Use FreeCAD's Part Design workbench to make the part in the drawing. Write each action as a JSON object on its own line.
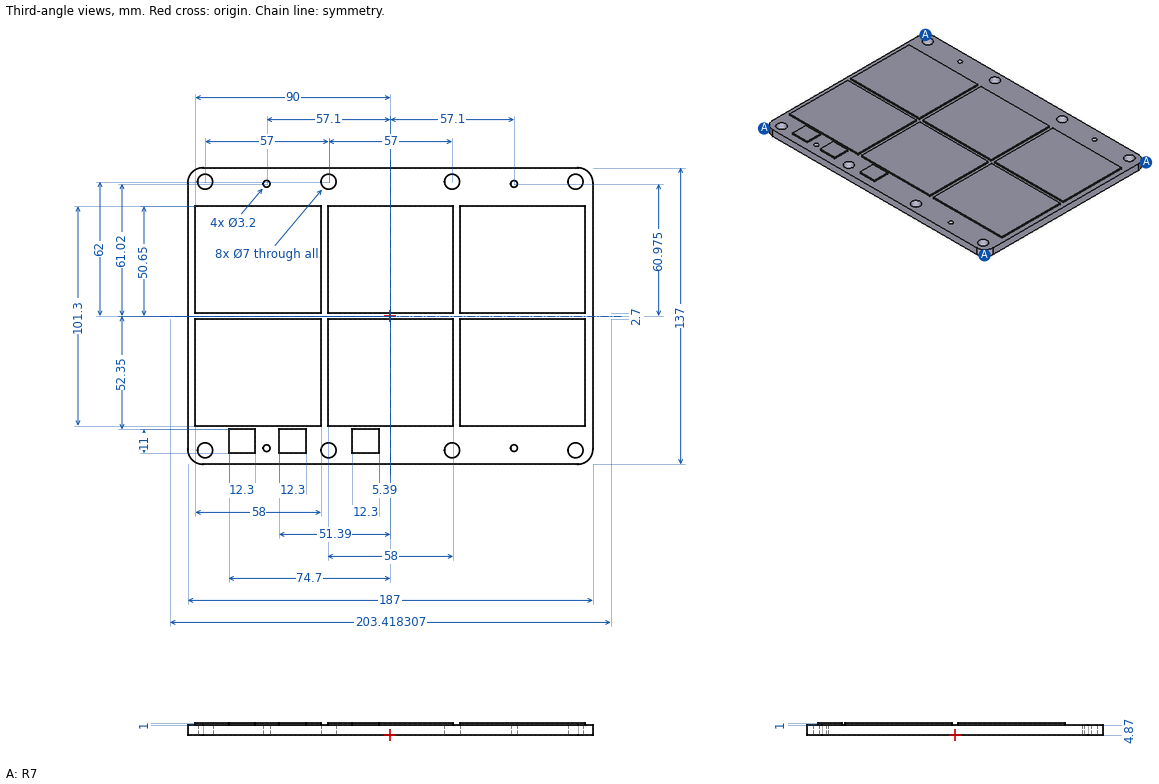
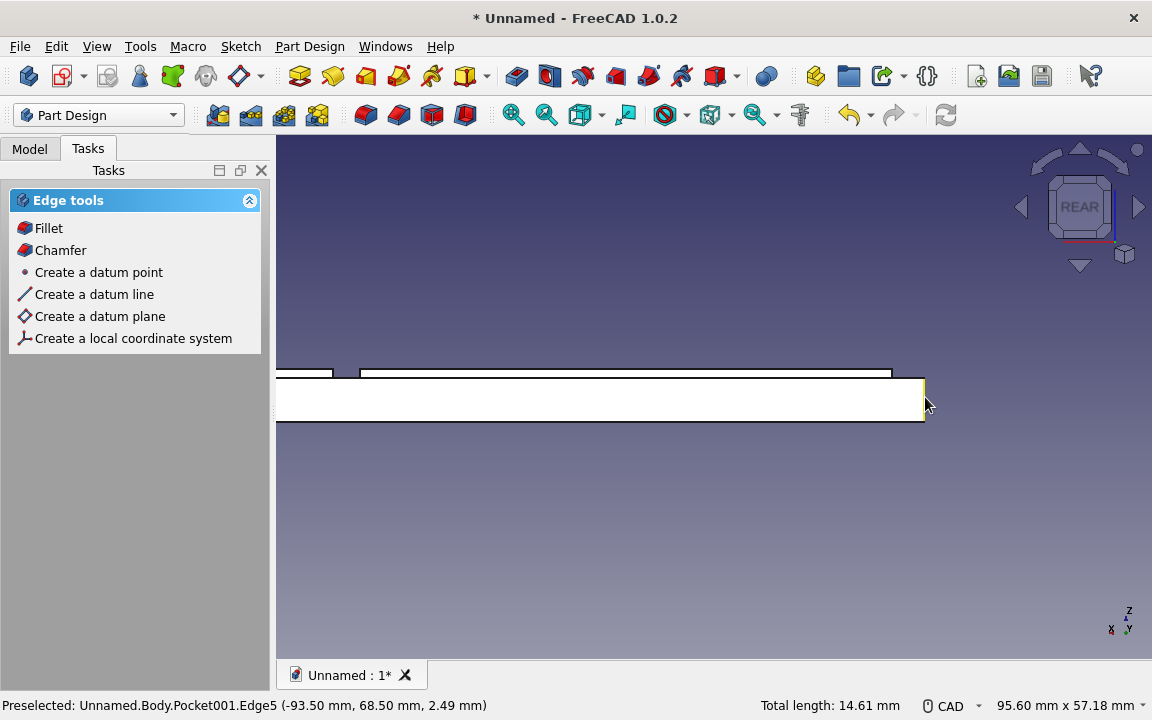
{"action": "left_click", "coordinate": [924, 399], "text": "ctrl"}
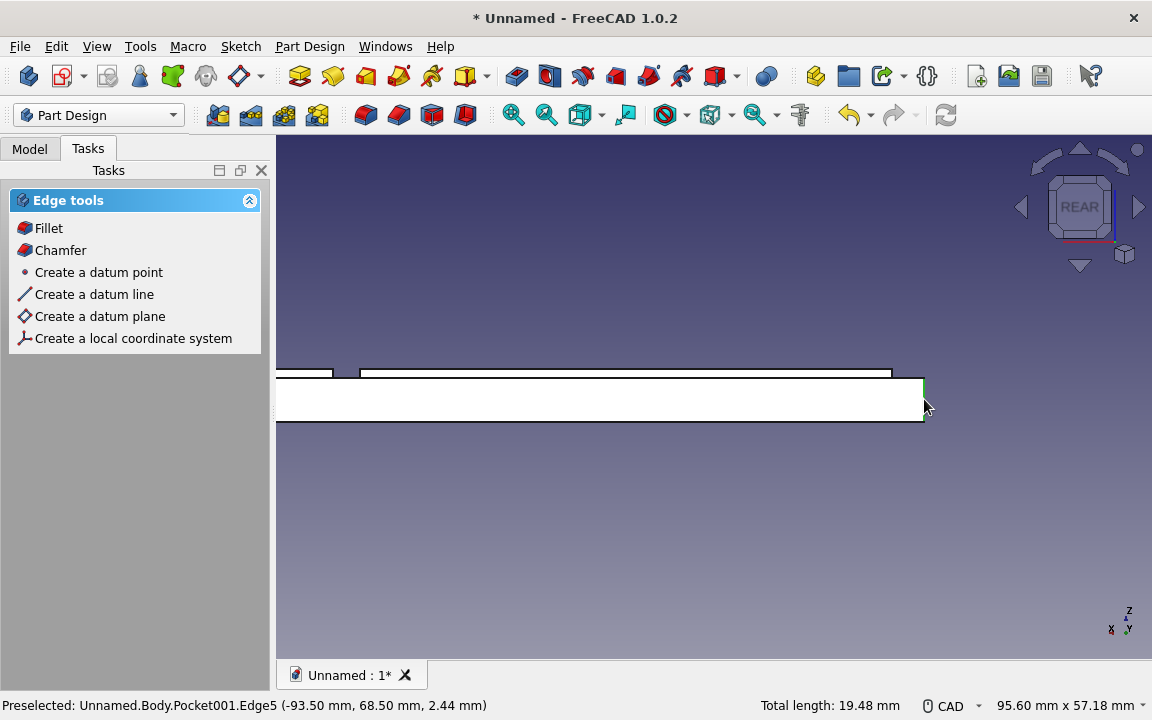
{"action": "left_click", "coordinate": [366, 116]}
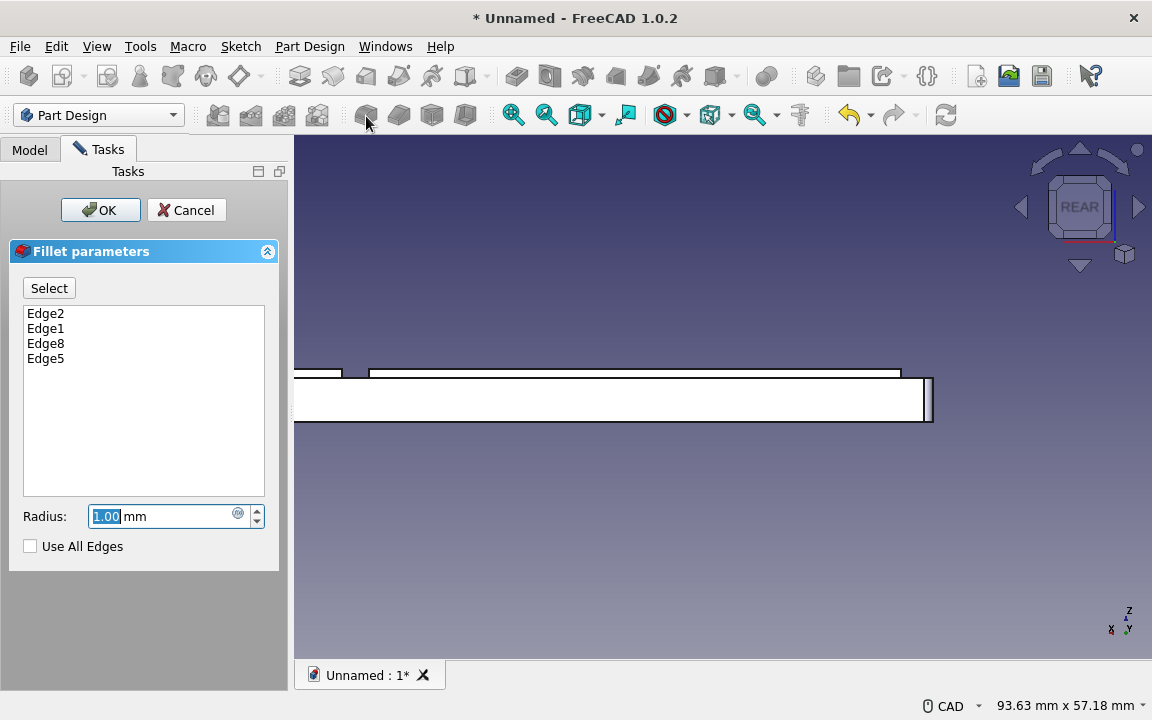
{"action": "type", "text": "7"}
{"action": "key", "text": "Tab"}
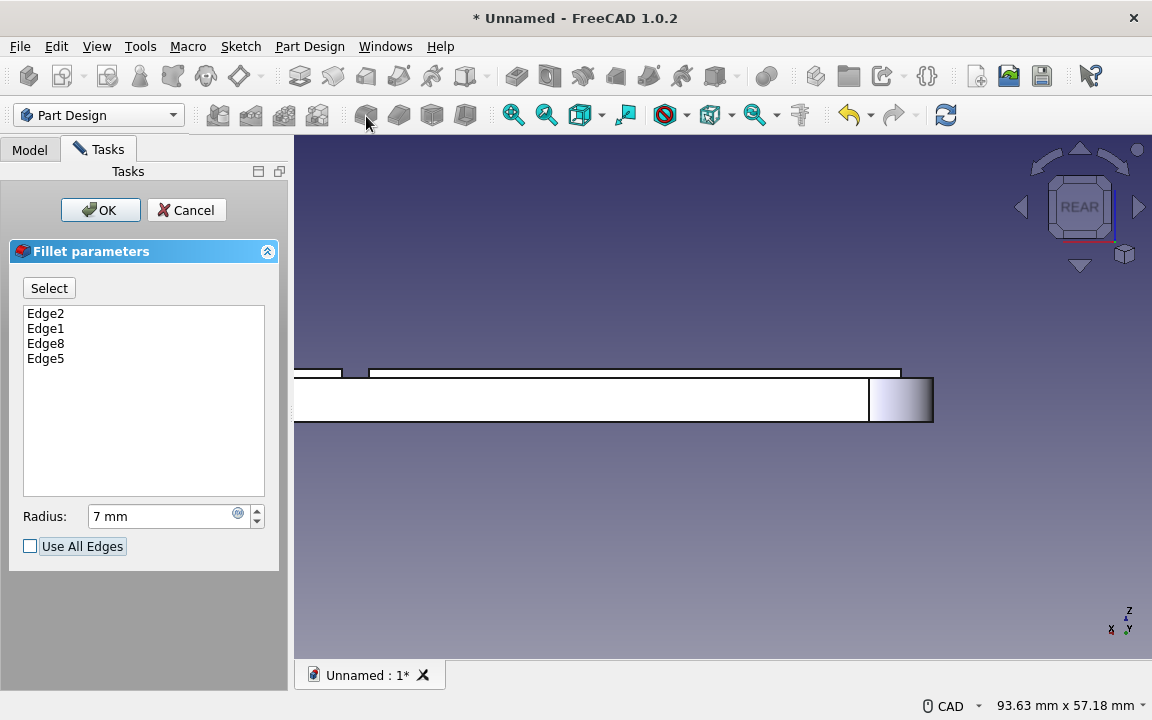
{"action": "left_click", "coordinate": [101, 210]}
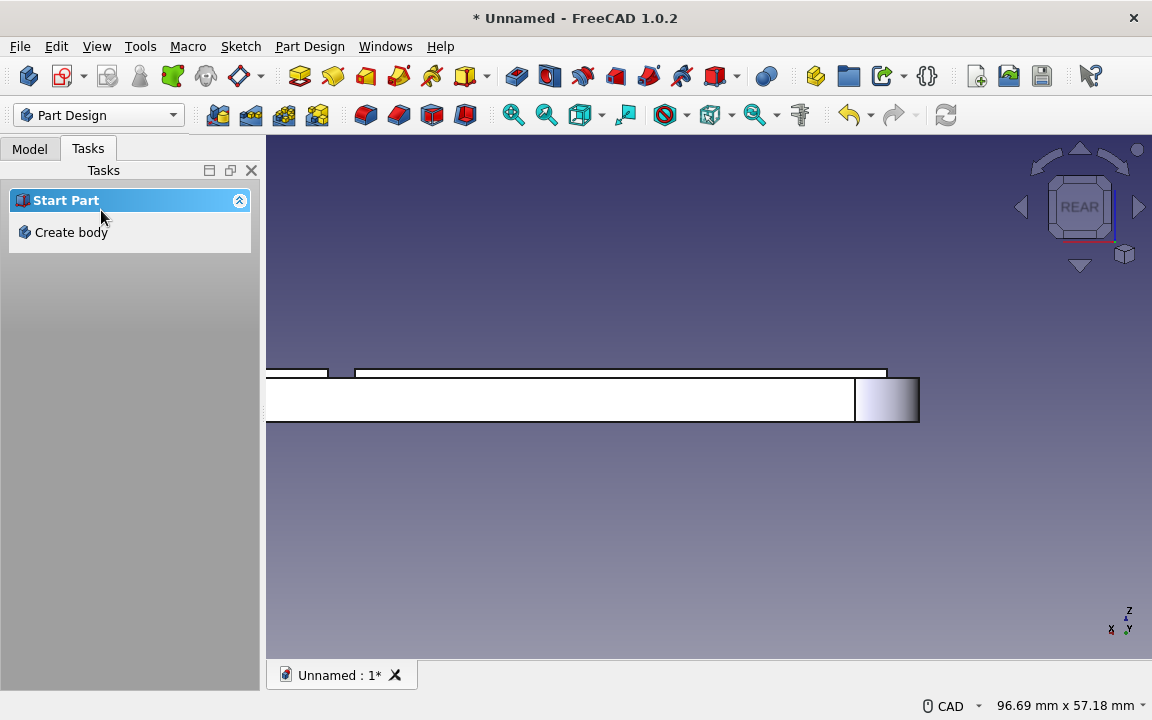
{"action": "key", "text": "0"}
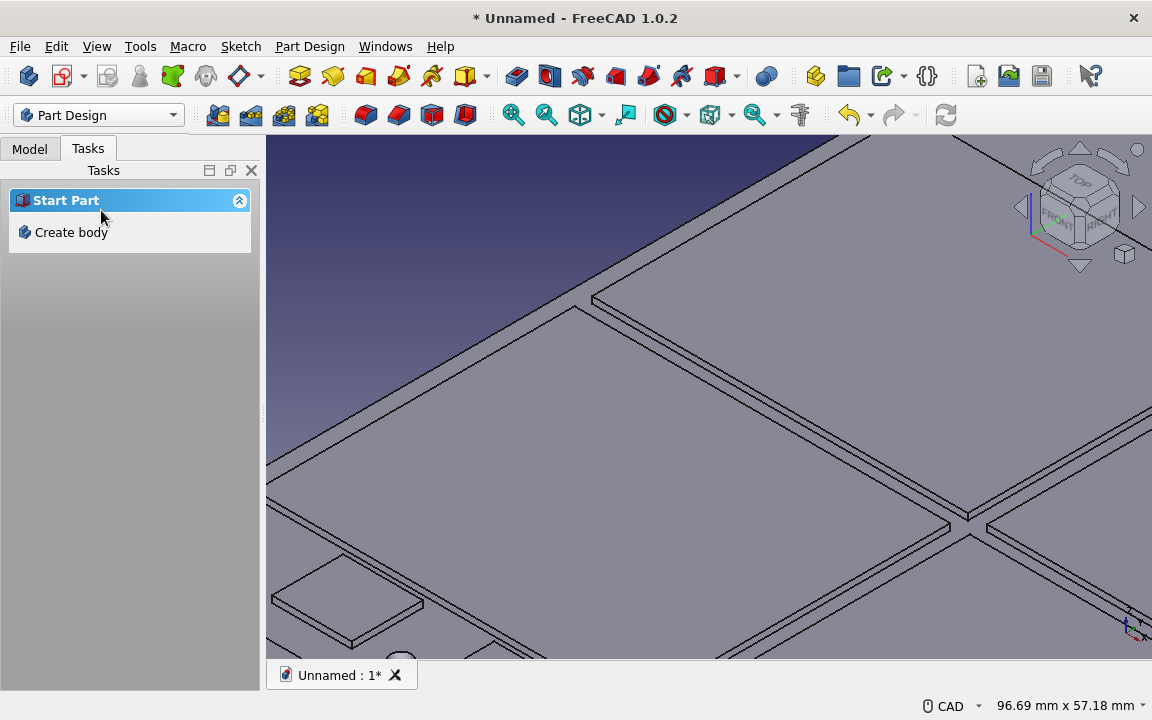
{"action": "key", "text": "v f"}